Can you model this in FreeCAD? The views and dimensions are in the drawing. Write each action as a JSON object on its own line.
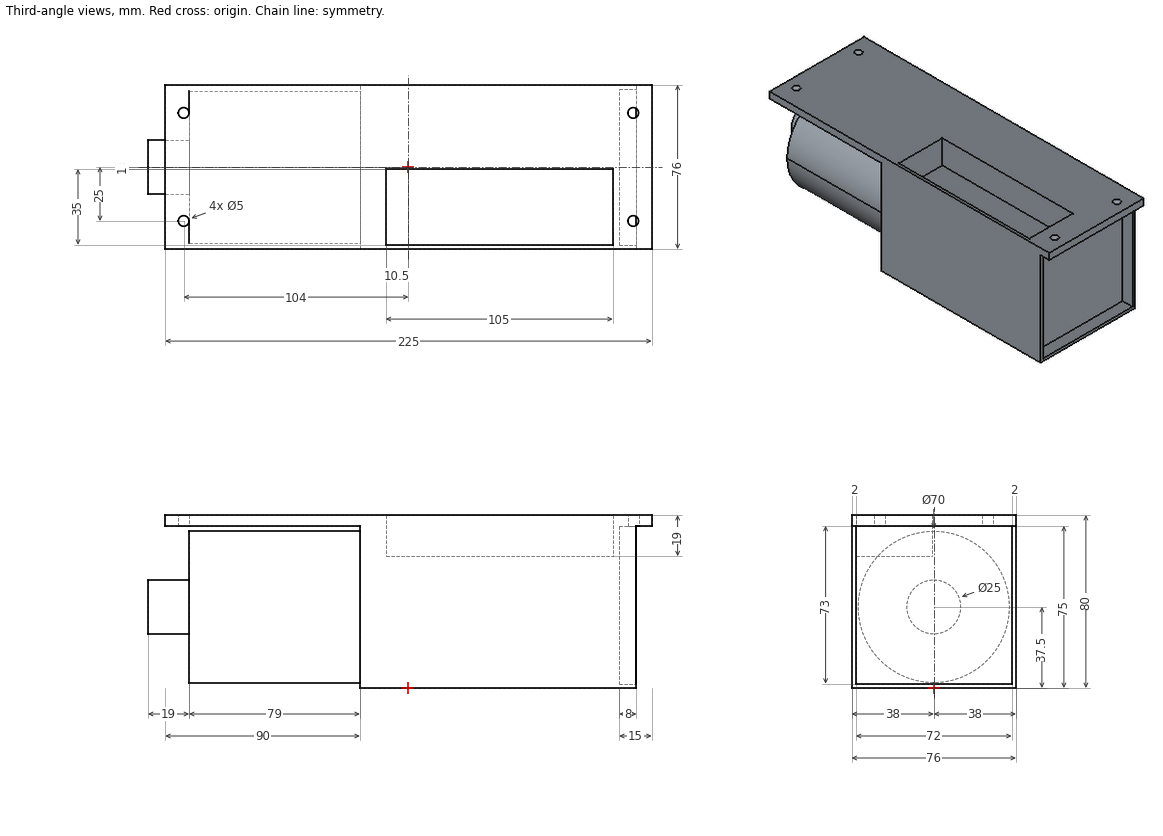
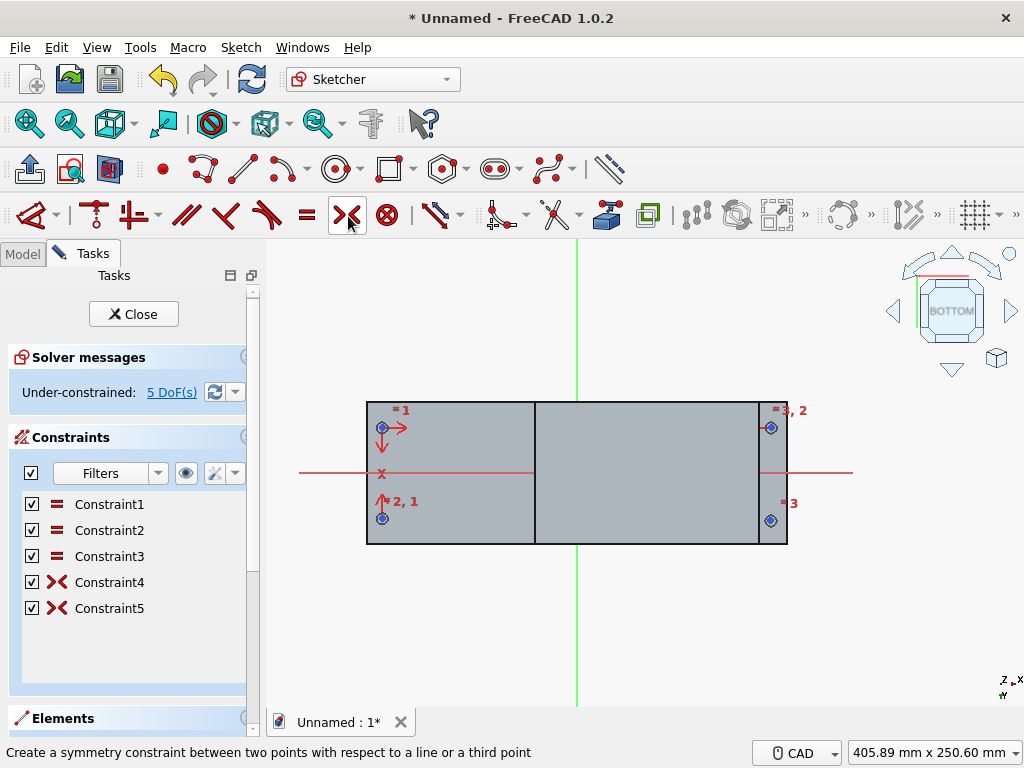
{"action": "left_click", "coordinate": [382, 519]}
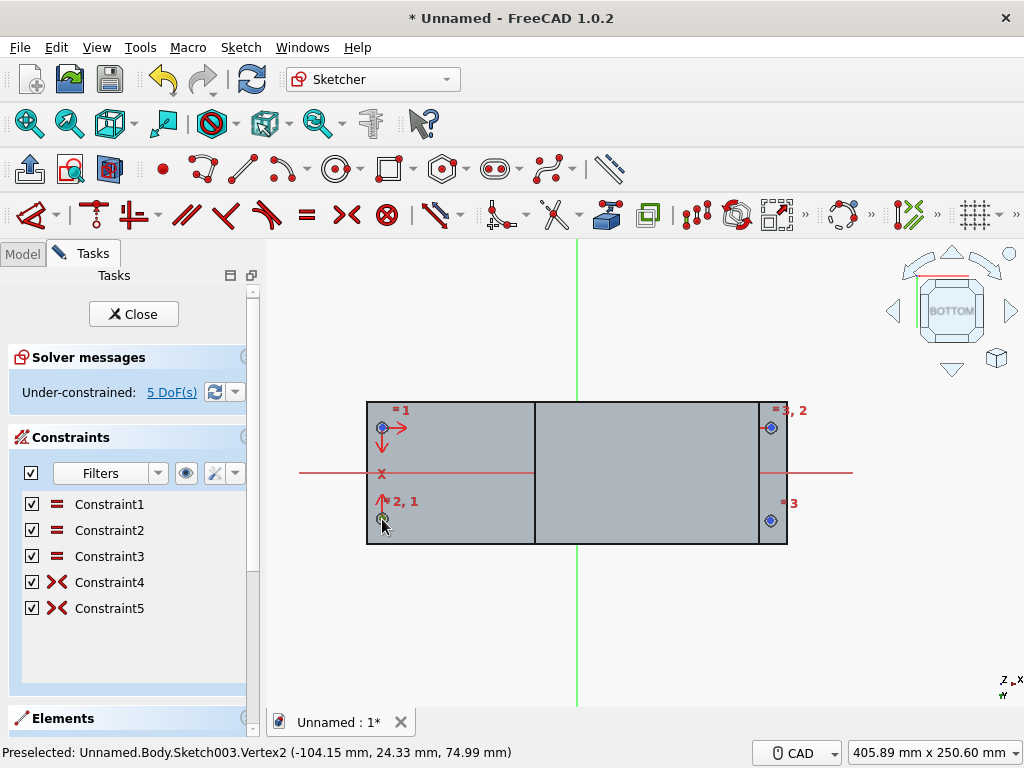
{"action": "left_click", "coordinate": [771, 521]}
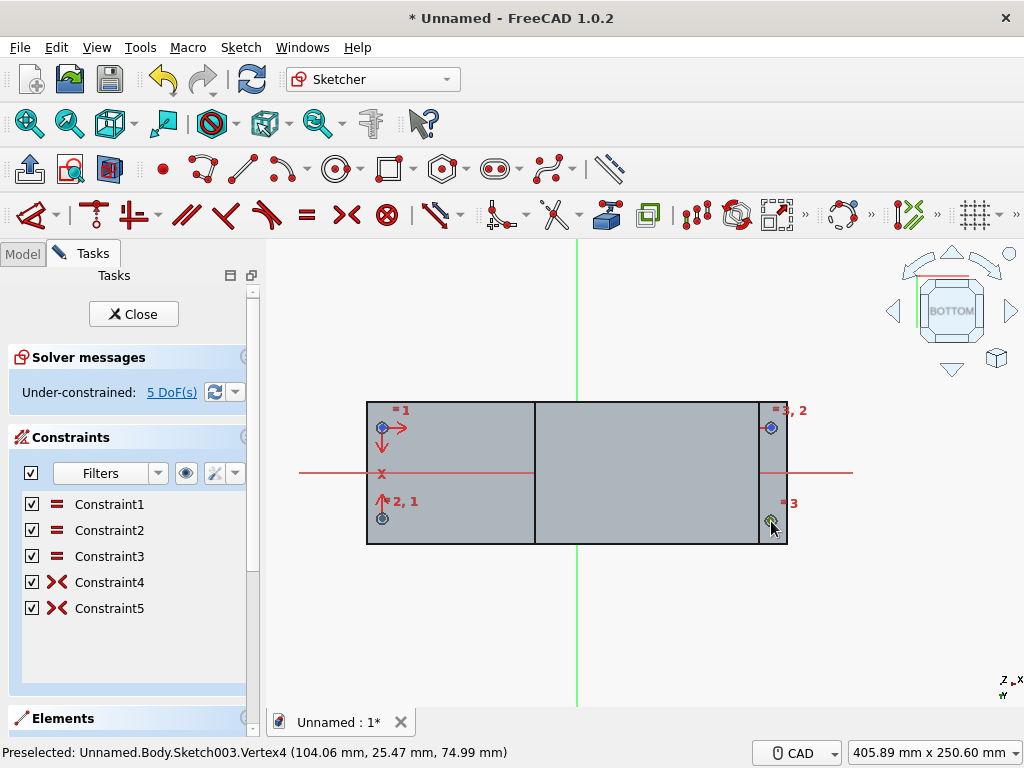
{"action": "left_click", "coordinate": [577, 650]}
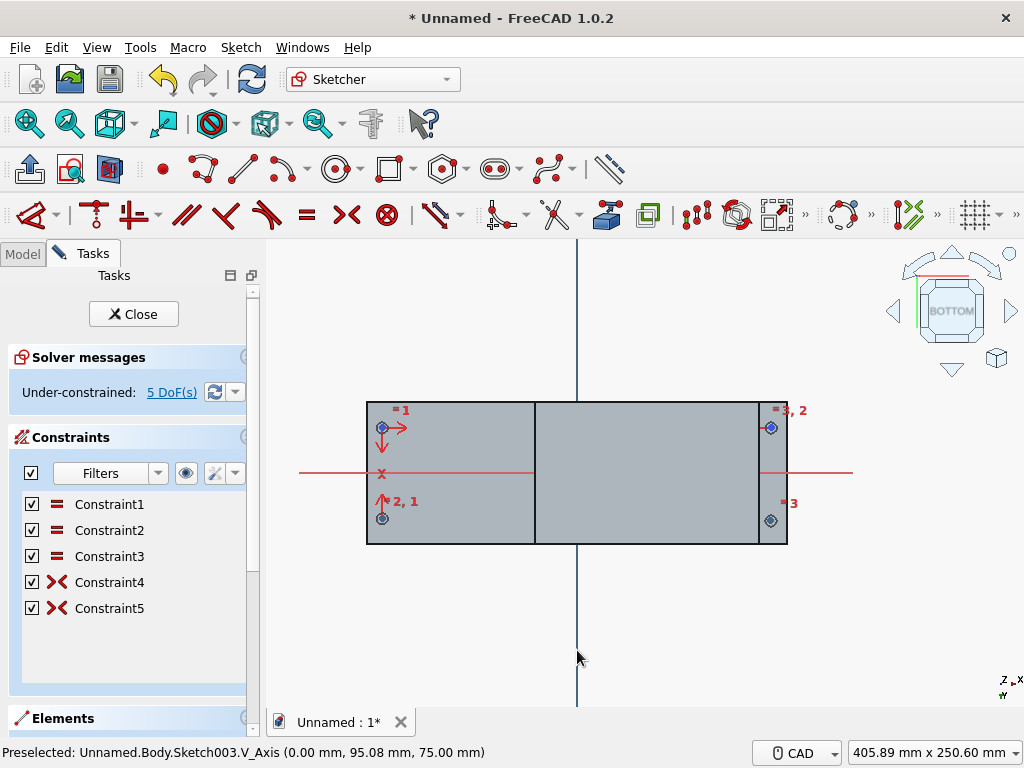
{"action": "key", "text": "s"}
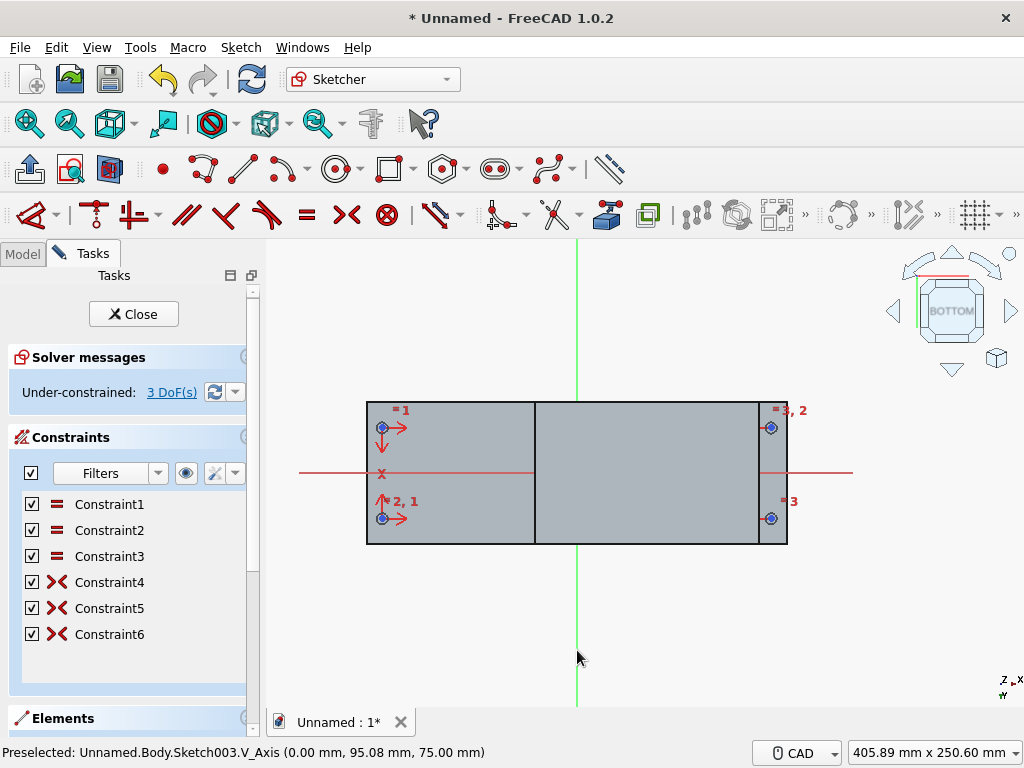
{"action": "key", "text": "d"}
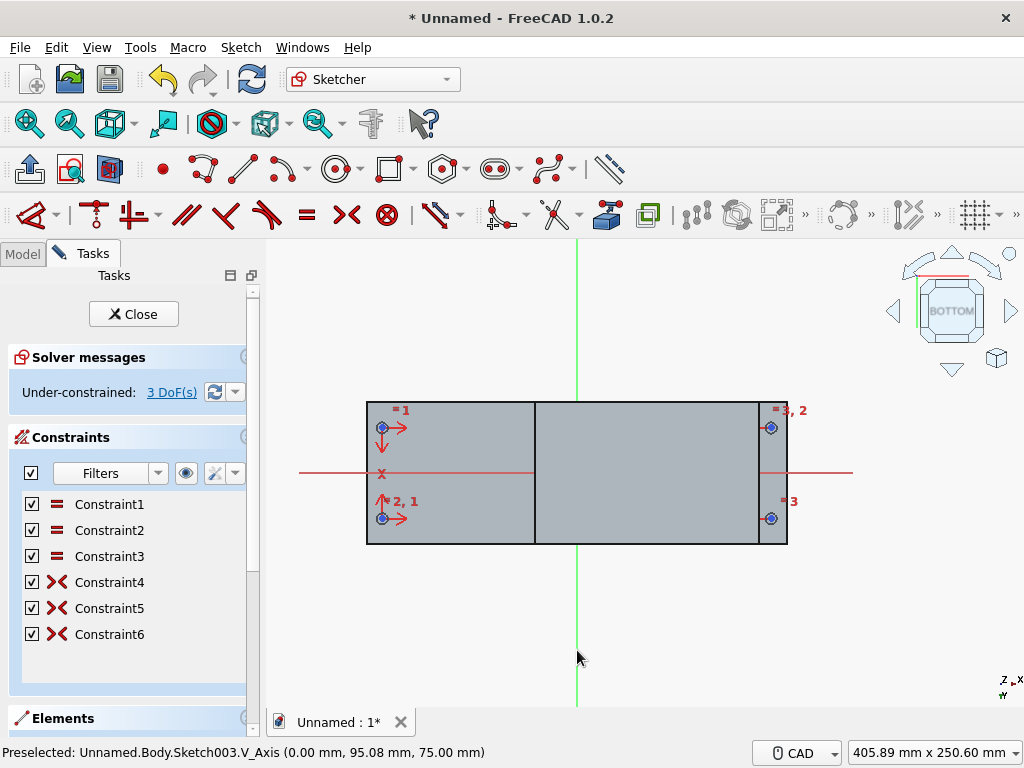
{"action": "scroll", "coordinate": [386, 424], "scroll_direction": "up", "scroll_amount": 8}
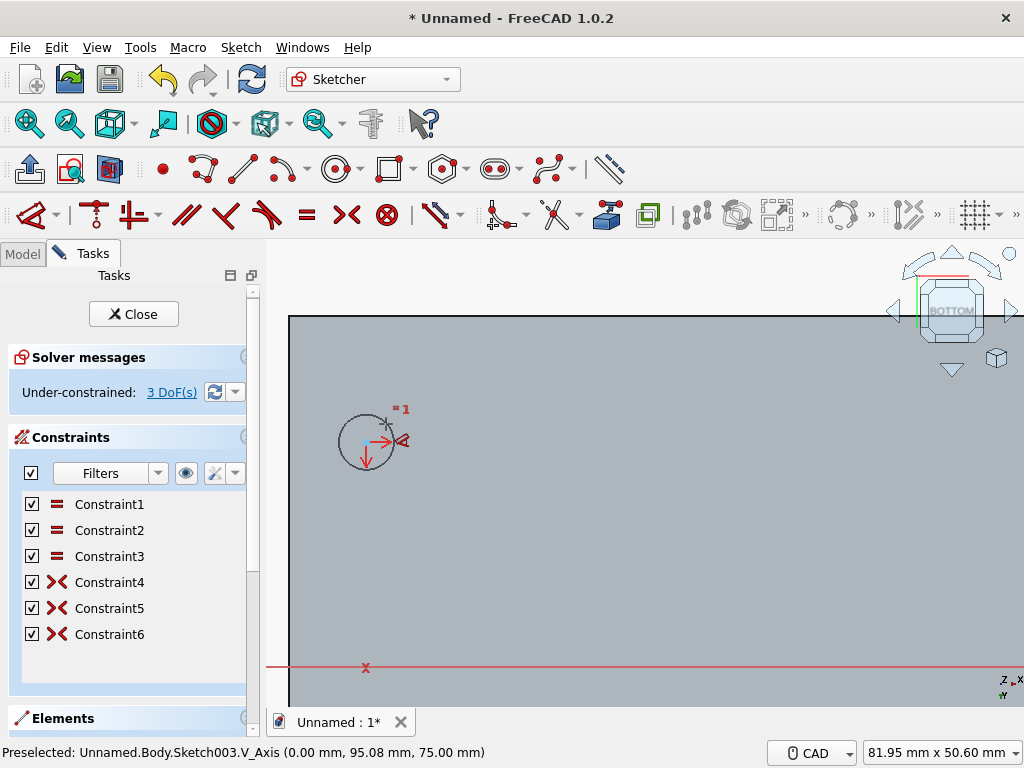
{"action": "left_click", "coordinate": [386, 423]}
{"action": "left_click", "coordinate": [409, 401]}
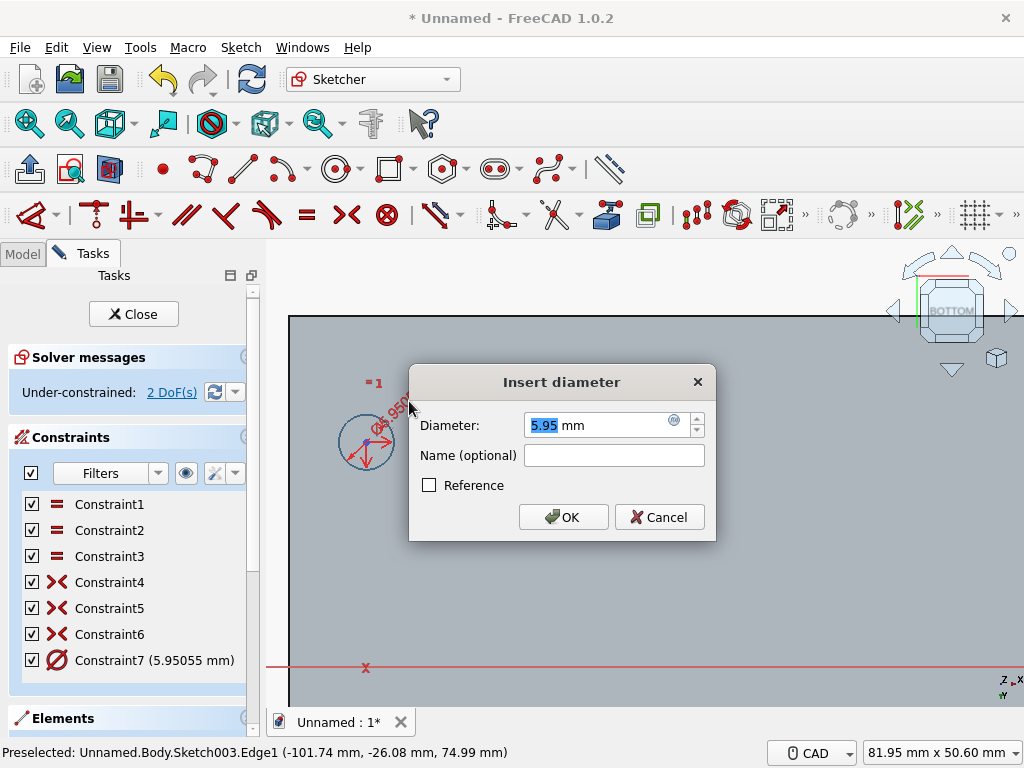
{"action": "type", "text": "5"}
{"action": "key", "text": "Return"}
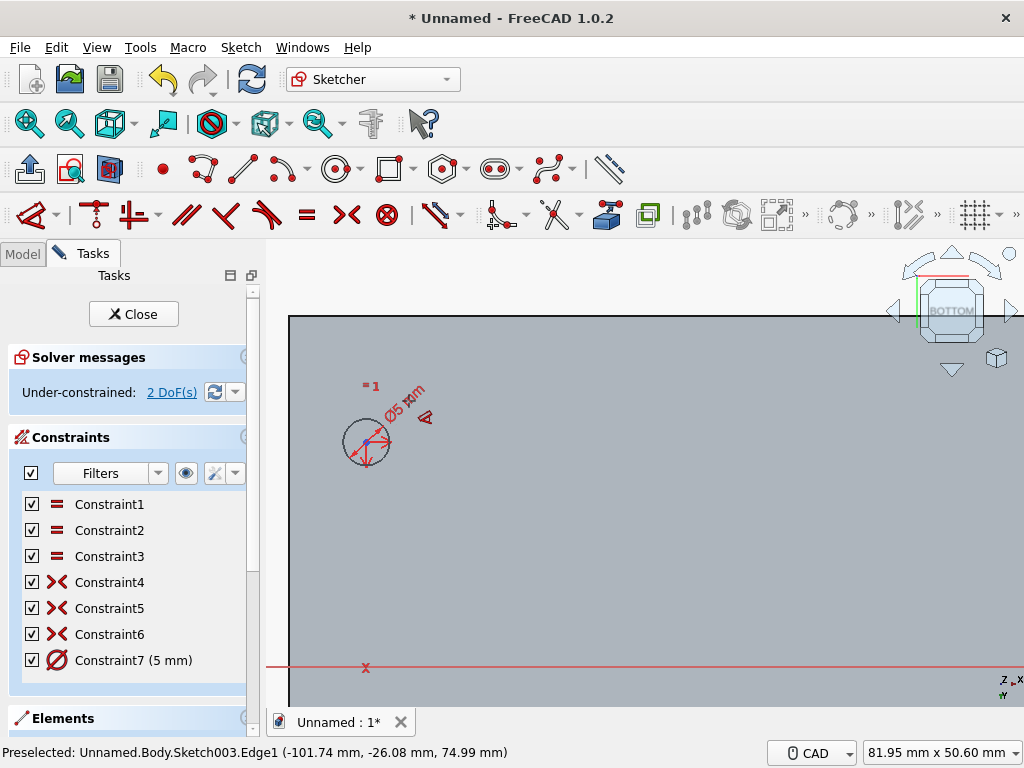
{"action": "scroll", "coordinate": [386, 424], "scroll_direction": "down", "scroll_amount": 8}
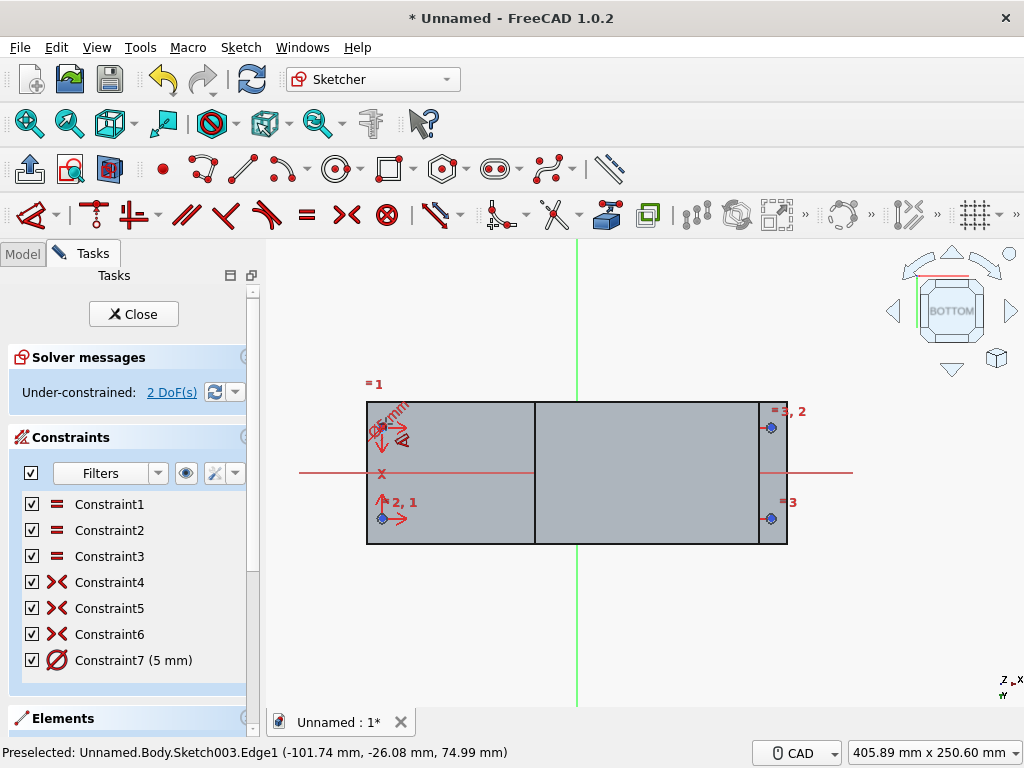
{"action": "left_click", "coordinate": [382, 428]}
{"action": "left_click", "coordinate": [348, 451]}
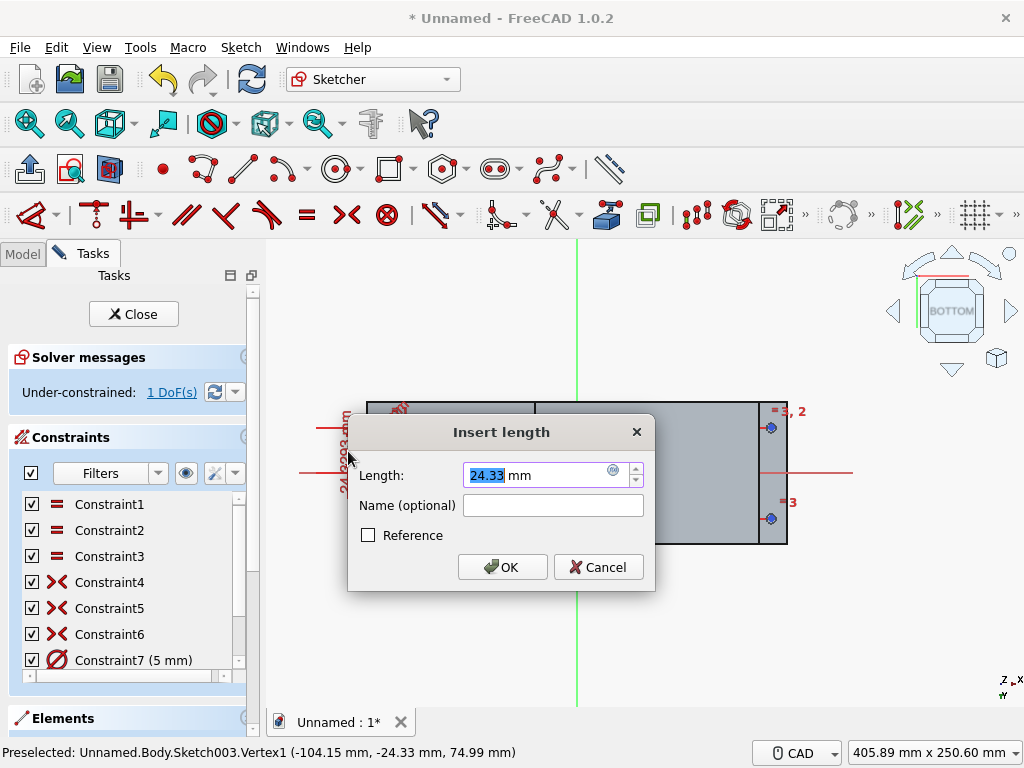
{"action": "type", "text": "25"}
{"action": "key", "text": "Return"}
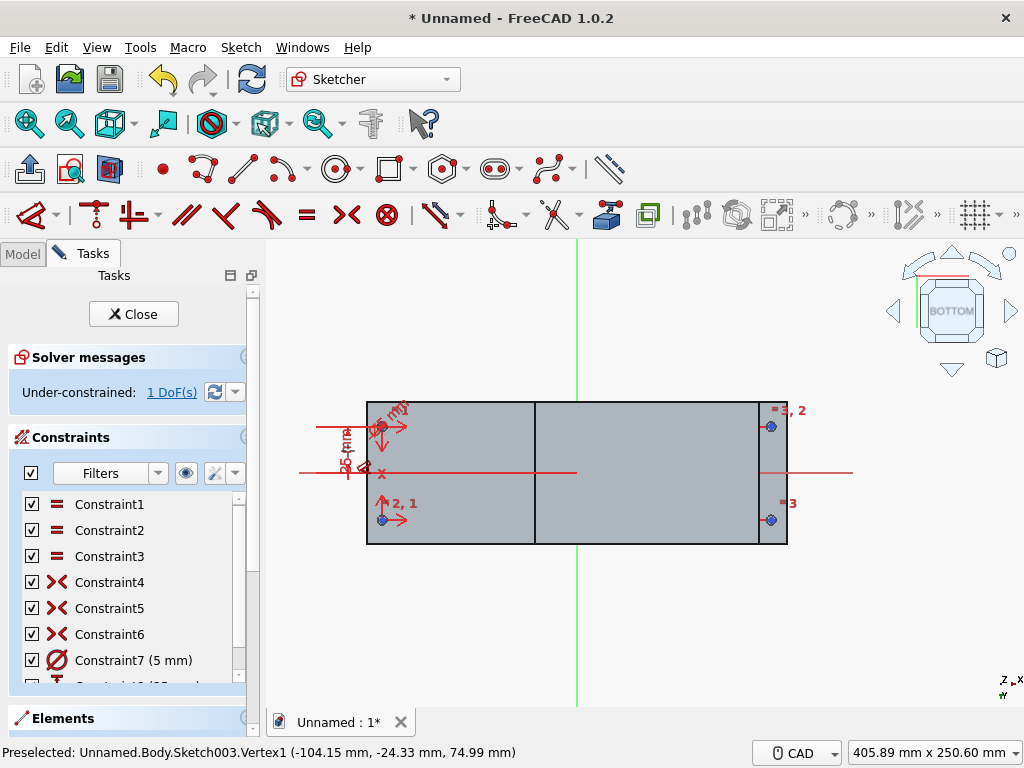
{"action": "left_click", "coordinate": [382, 427]}
{"action": "left_click", "coordinate": [479, 393]}